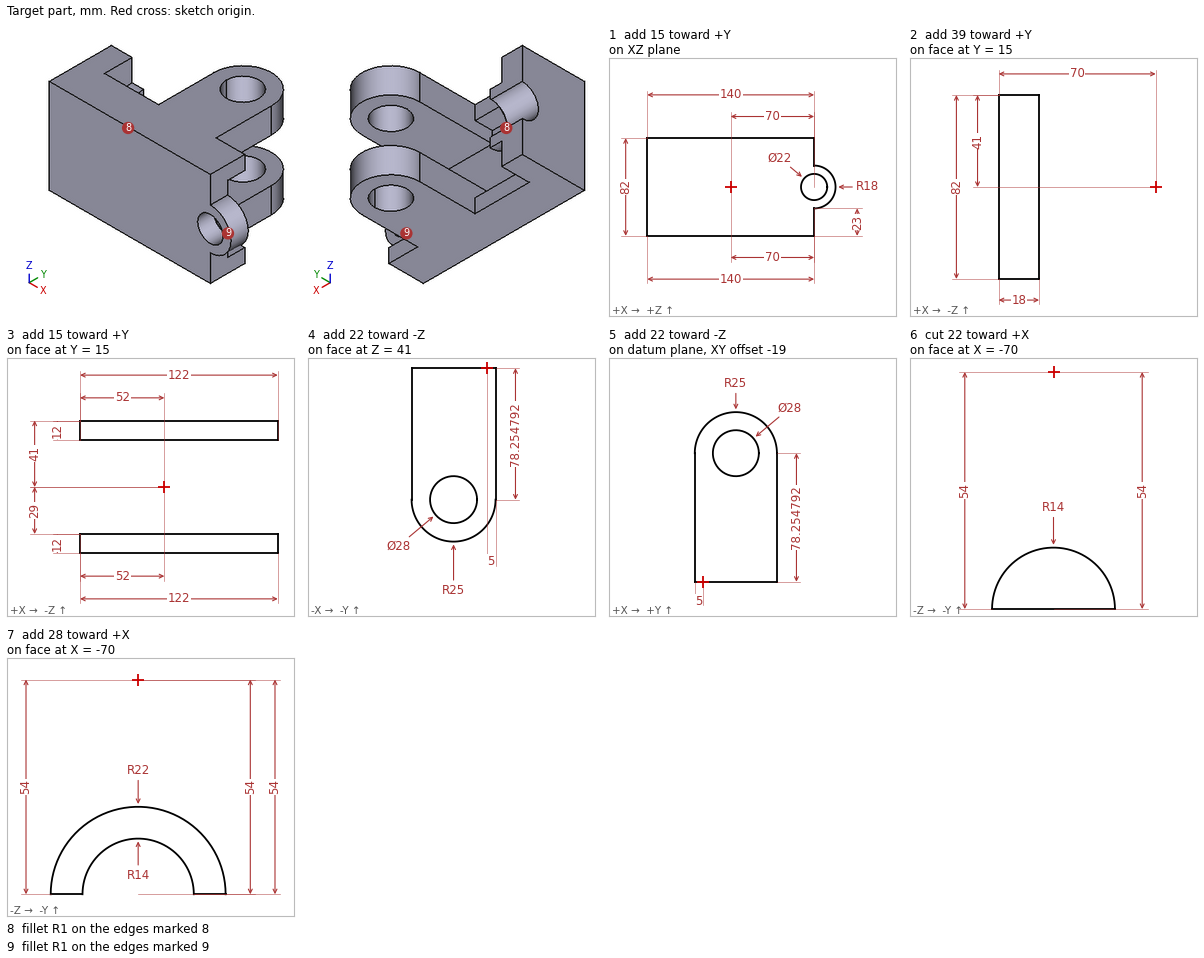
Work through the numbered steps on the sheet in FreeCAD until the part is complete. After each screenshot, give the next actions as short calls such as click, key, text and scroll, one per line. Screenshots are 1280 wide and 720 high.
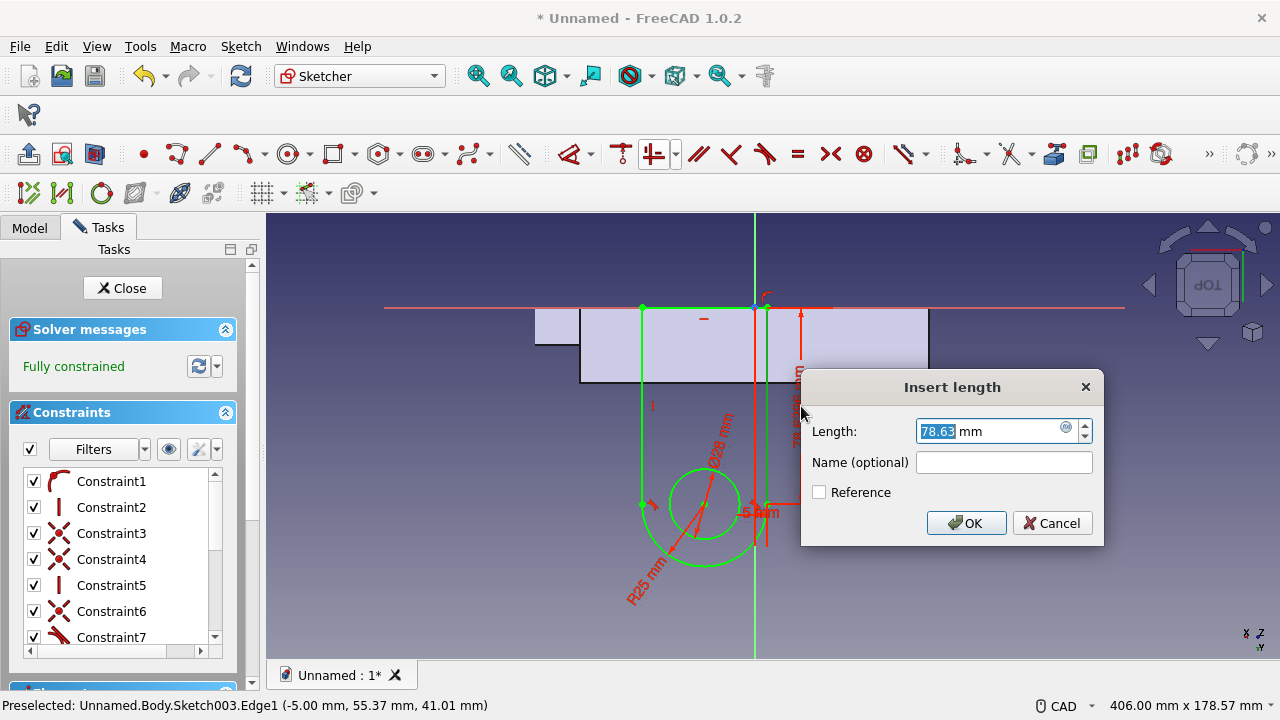
text(78.254792)
key(Return)
key(Escape)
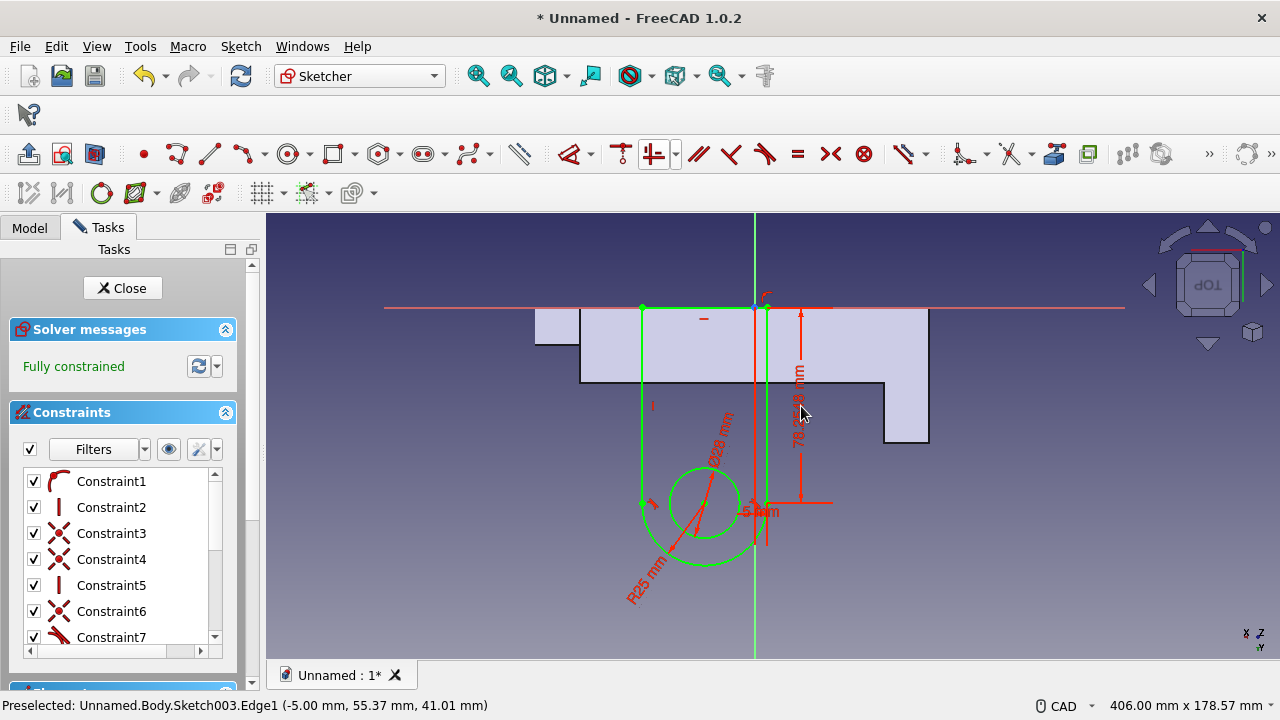
click(123, 288)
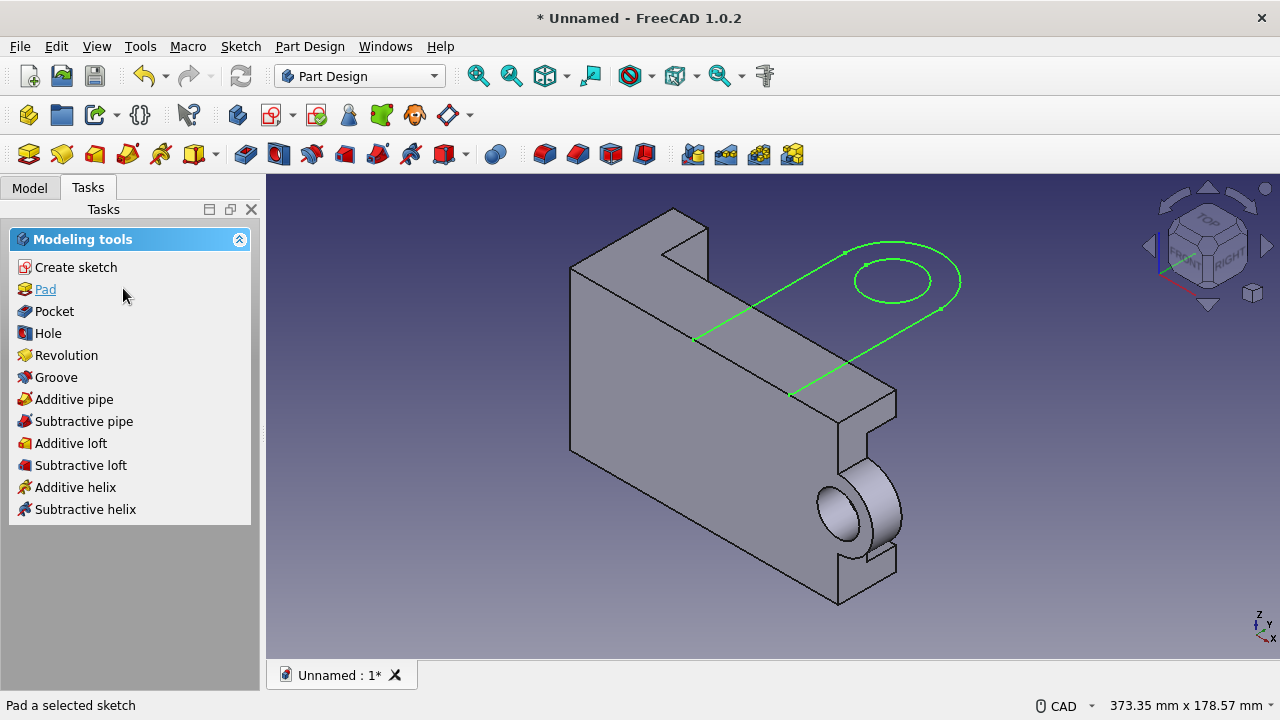
click(29, 154)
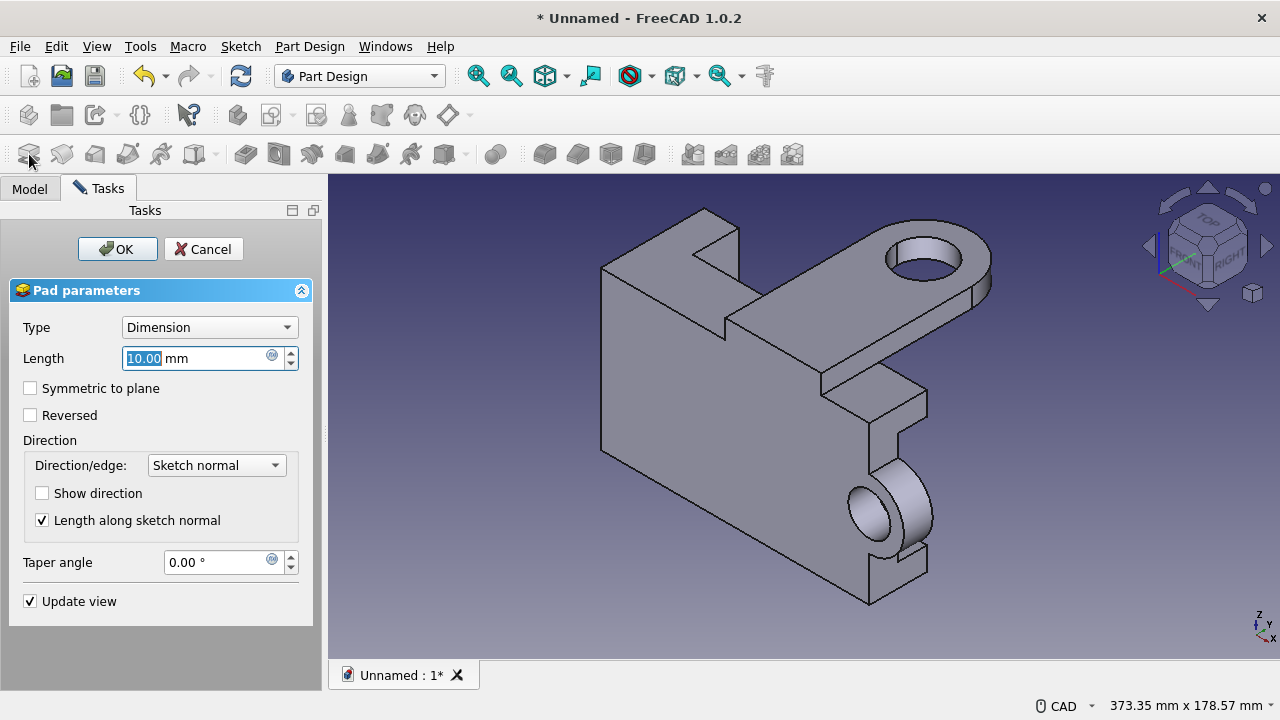
text(22)
key(Tab)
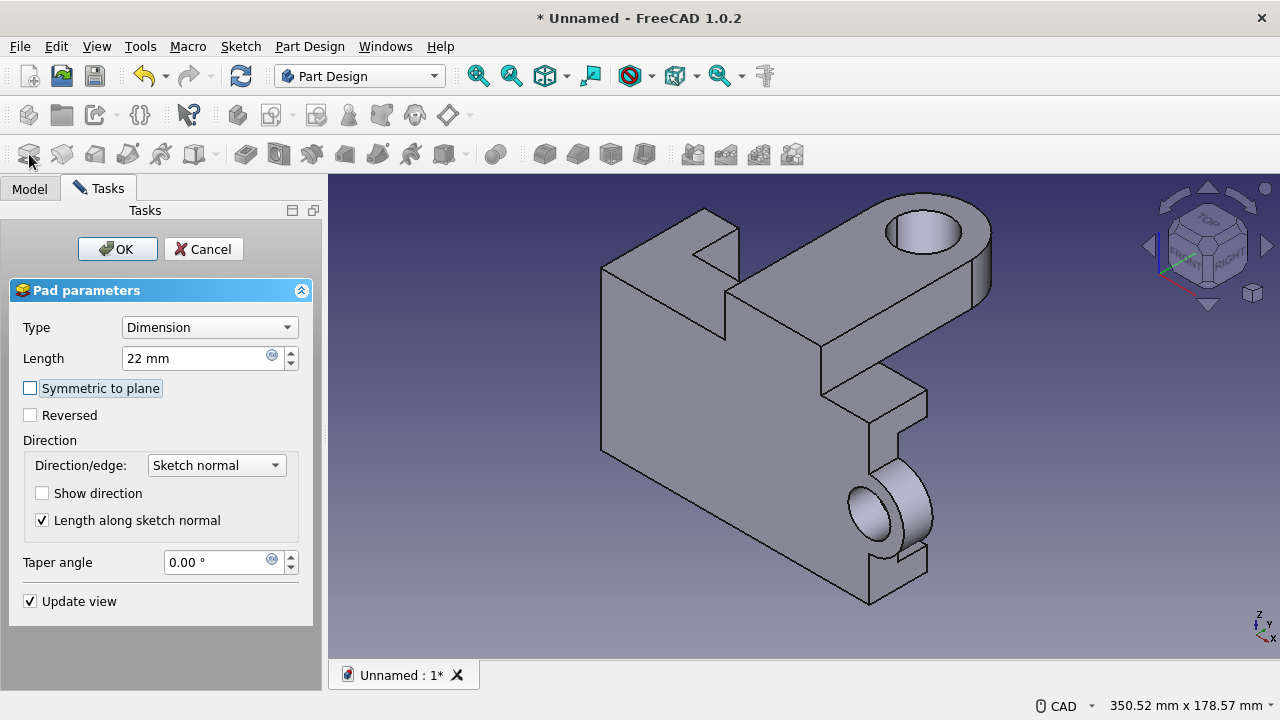
click(31, 415)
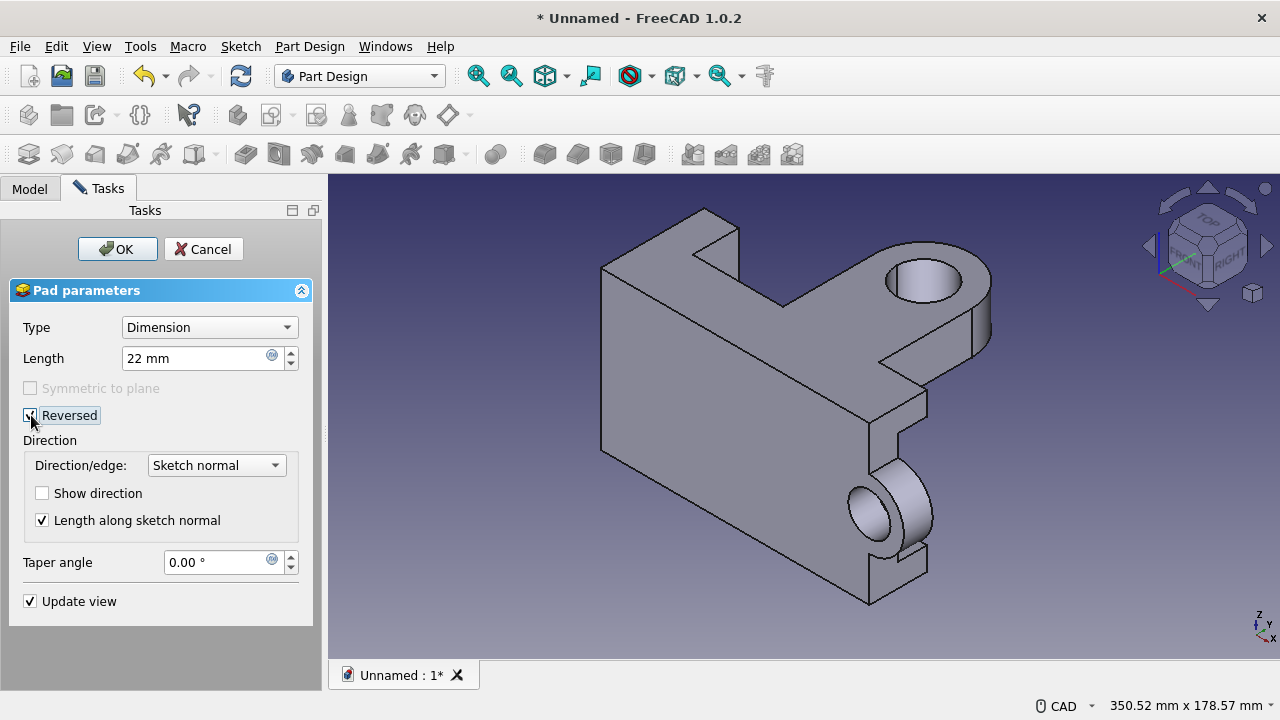
click(118, 249)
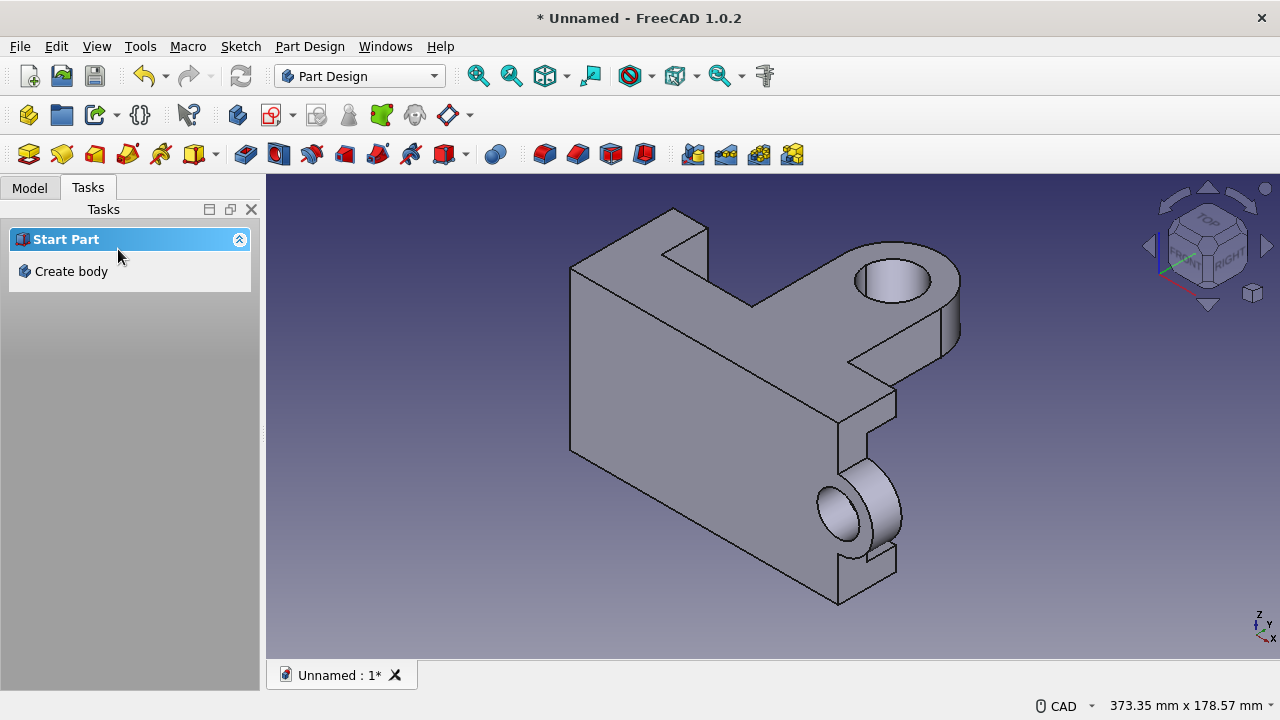
click(479, 76)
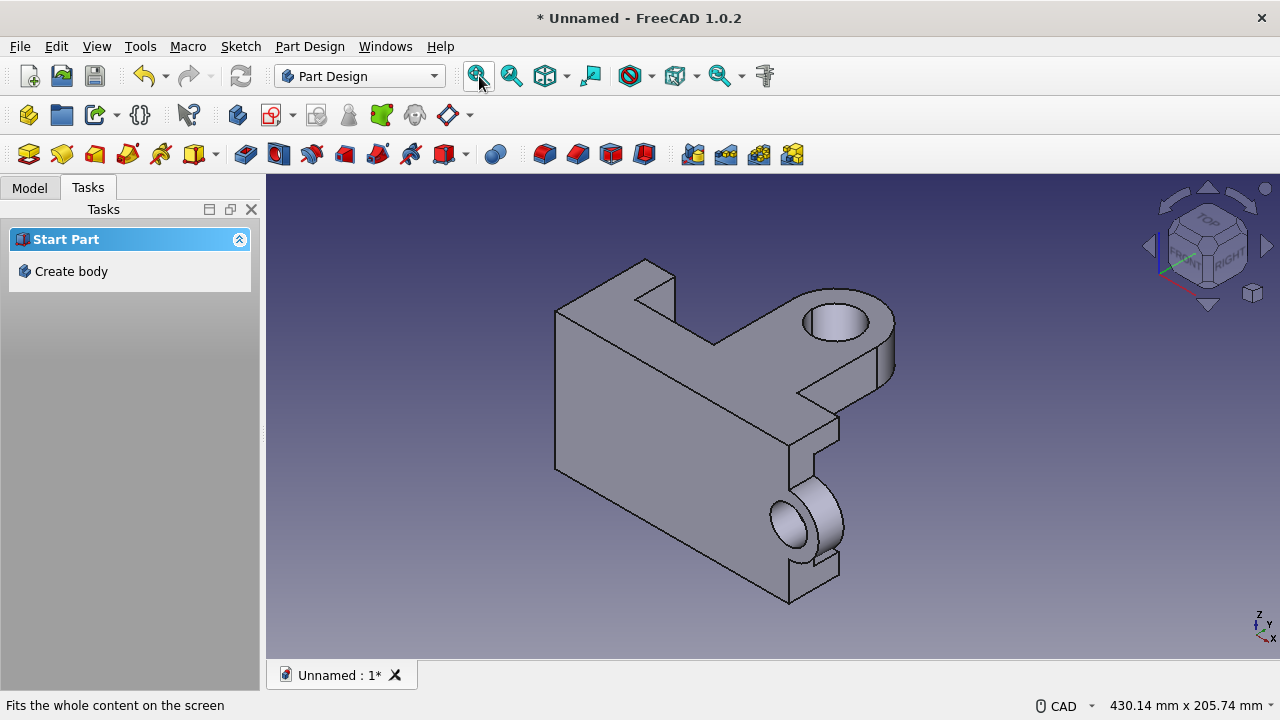
click(30, 188)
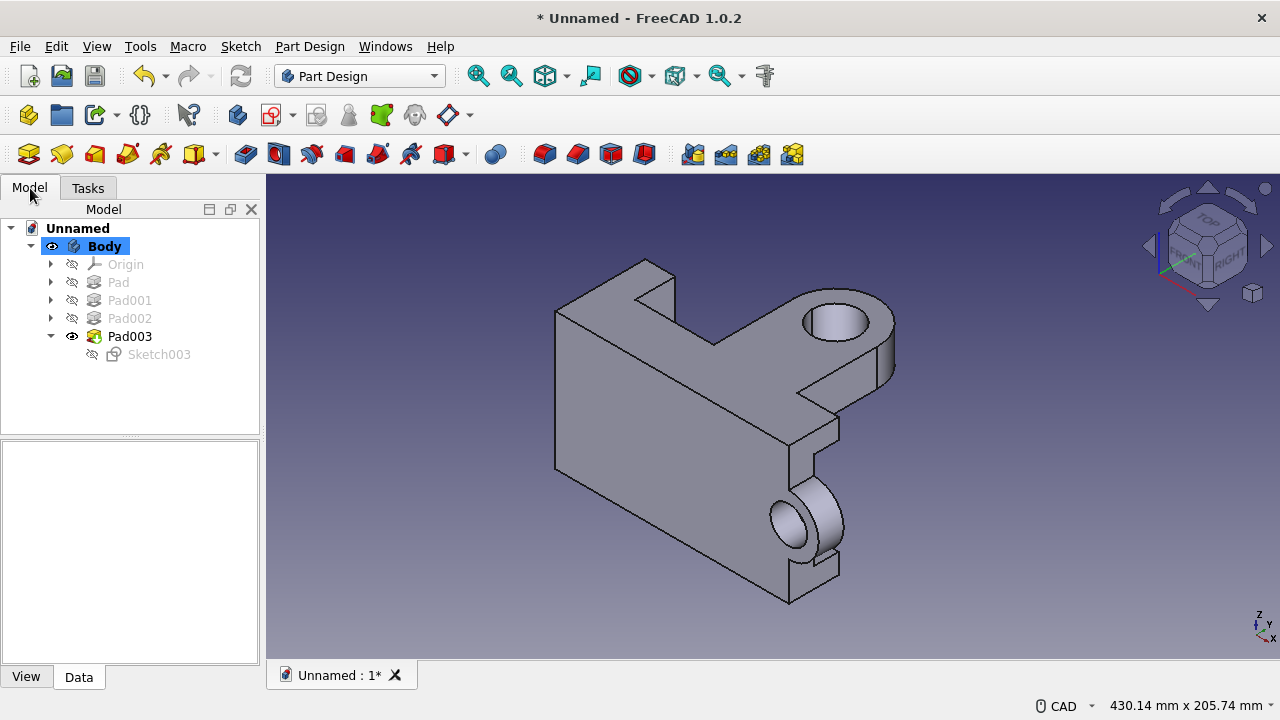
click(51, 264)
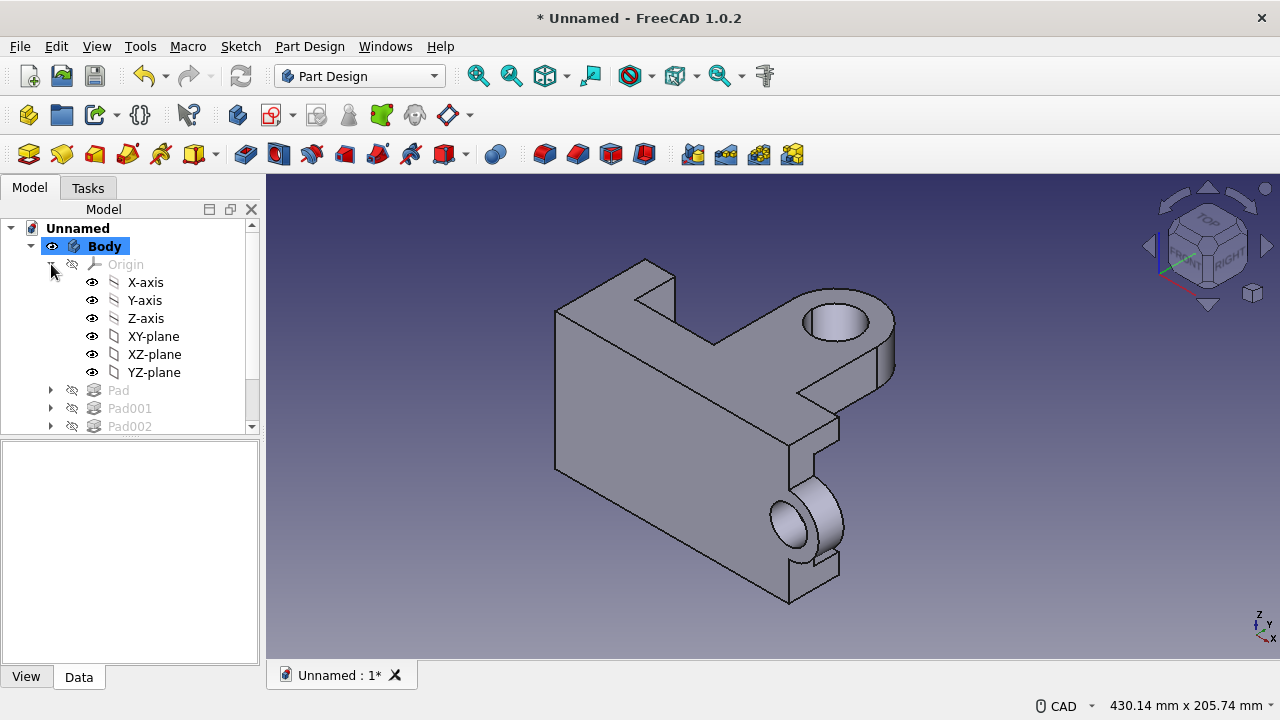
click(137, 336)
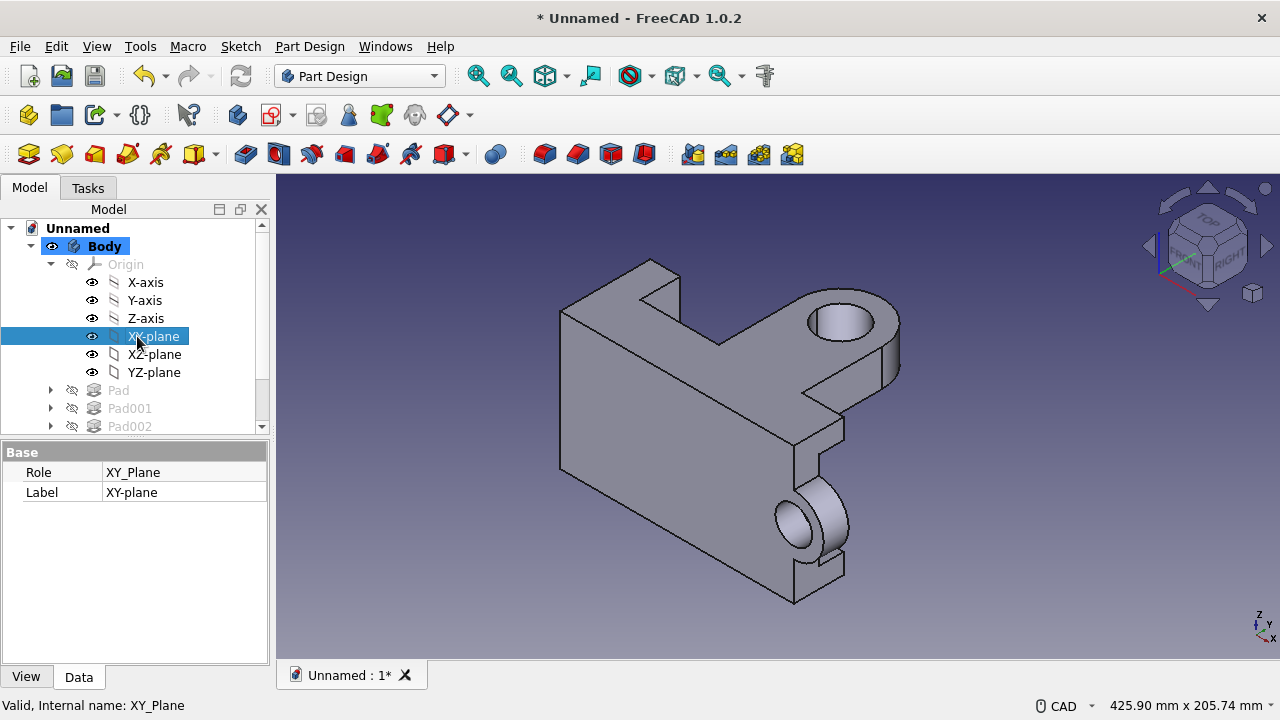
click(448, 116)